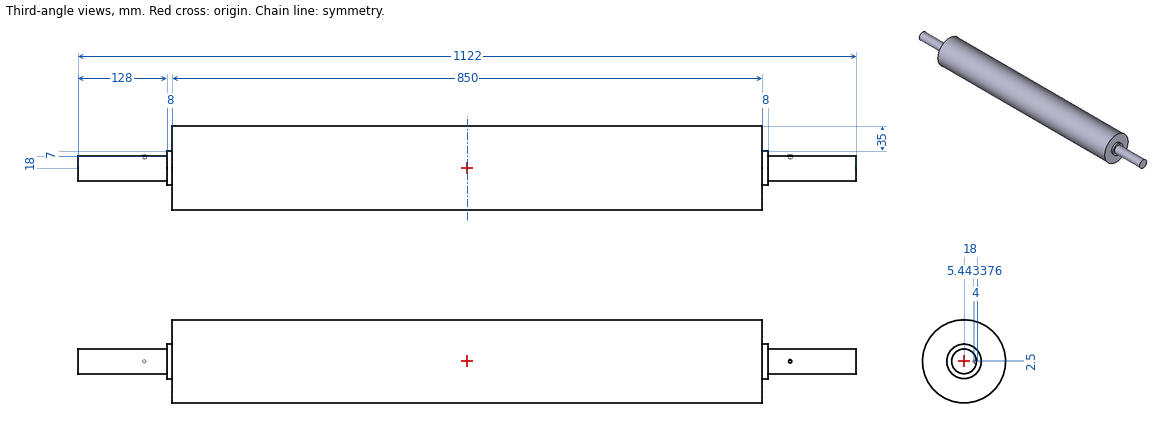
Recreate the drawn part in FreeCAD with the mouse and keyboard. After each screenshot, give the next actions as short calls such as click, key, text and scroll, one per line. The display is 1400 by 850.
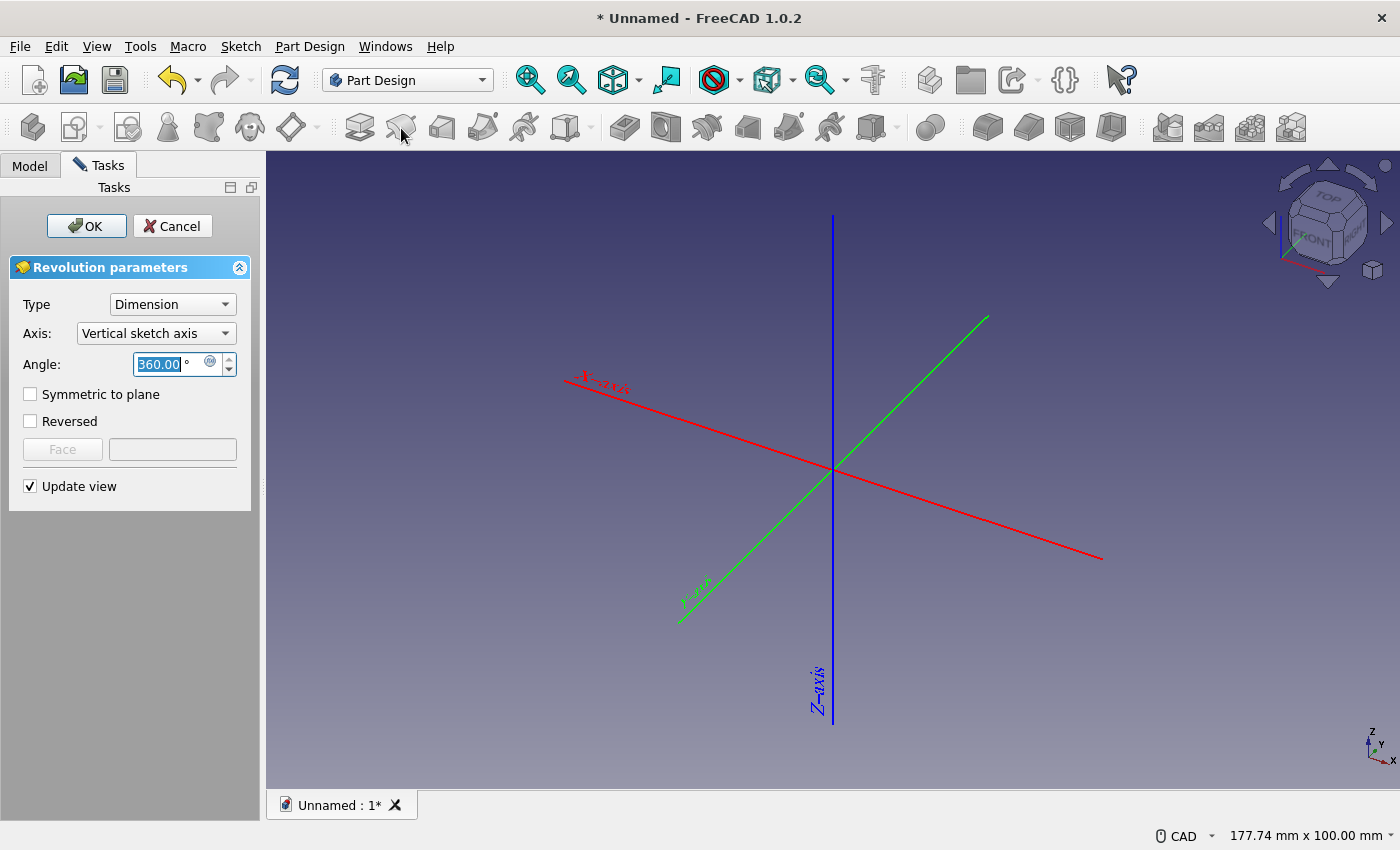
click(157, 334)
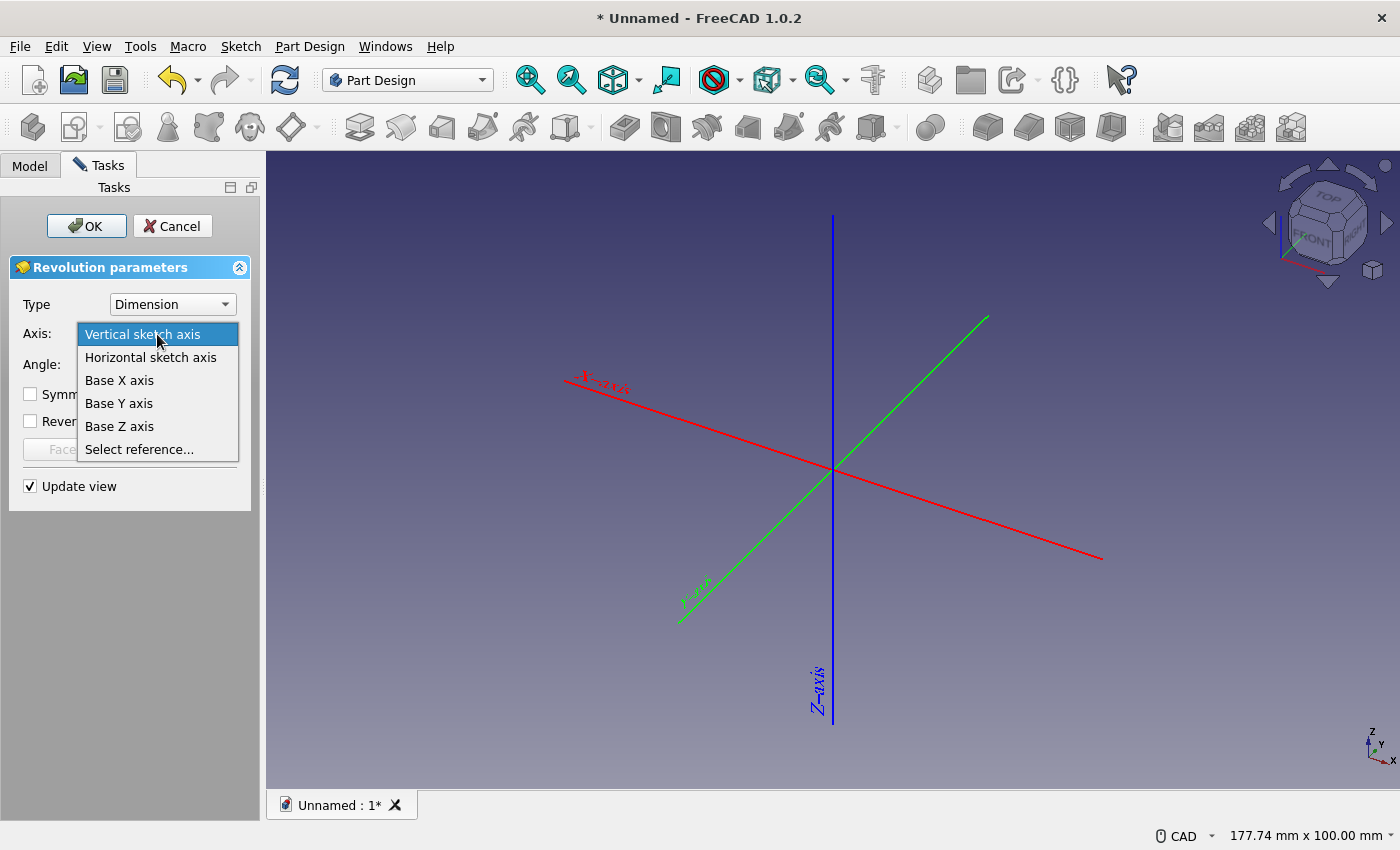
click(156, 358)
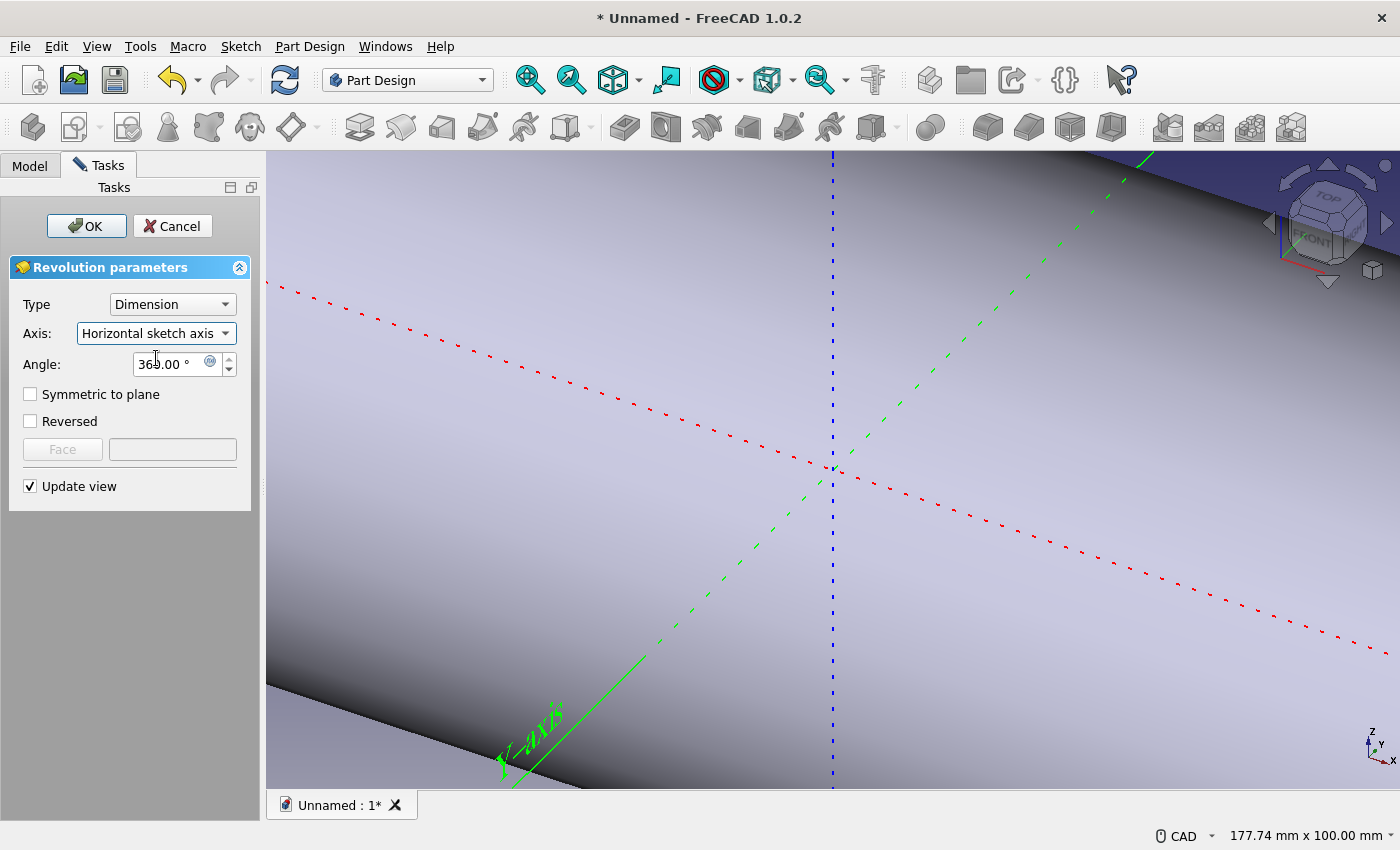
click(87, 226)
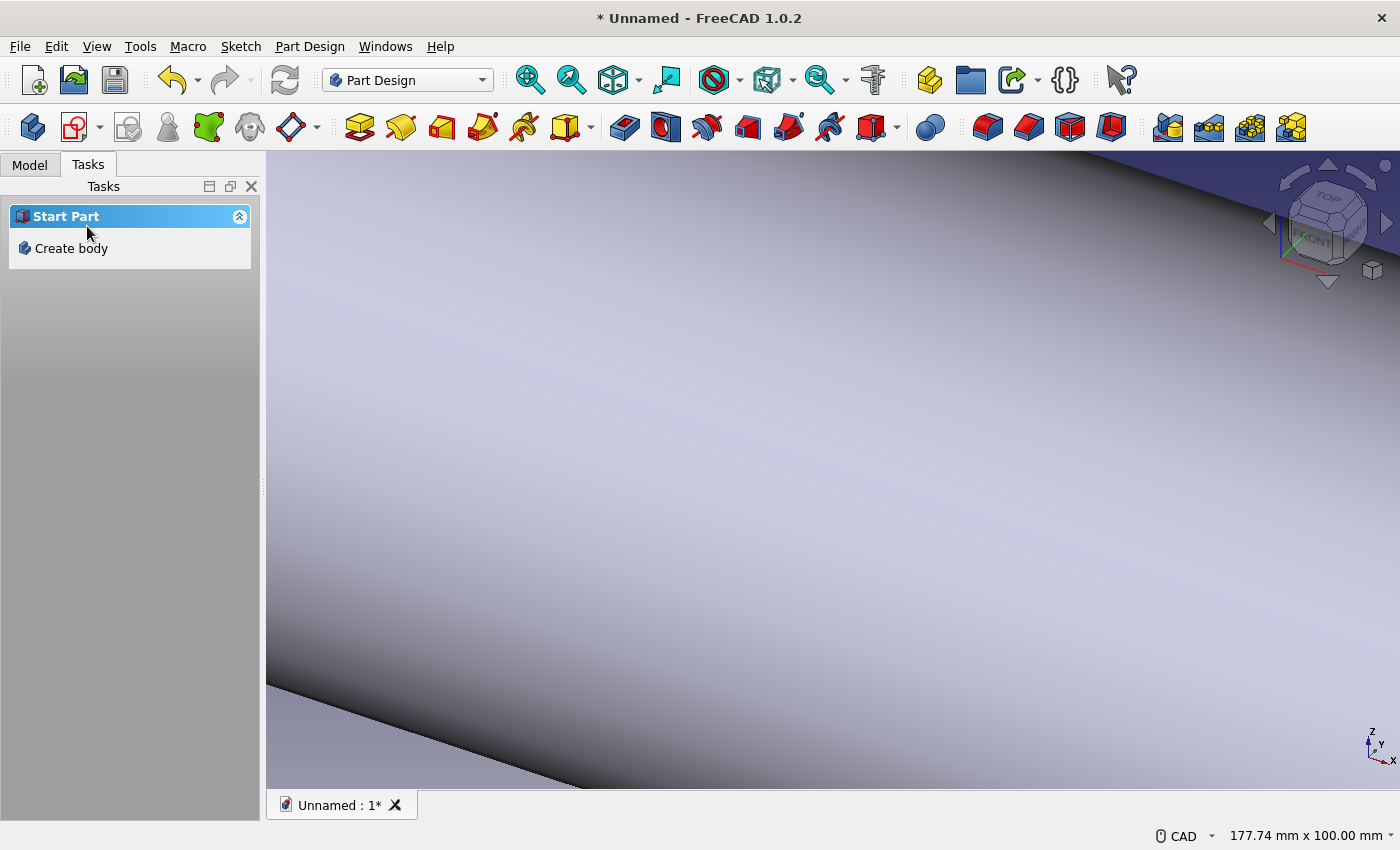
click(531, 80)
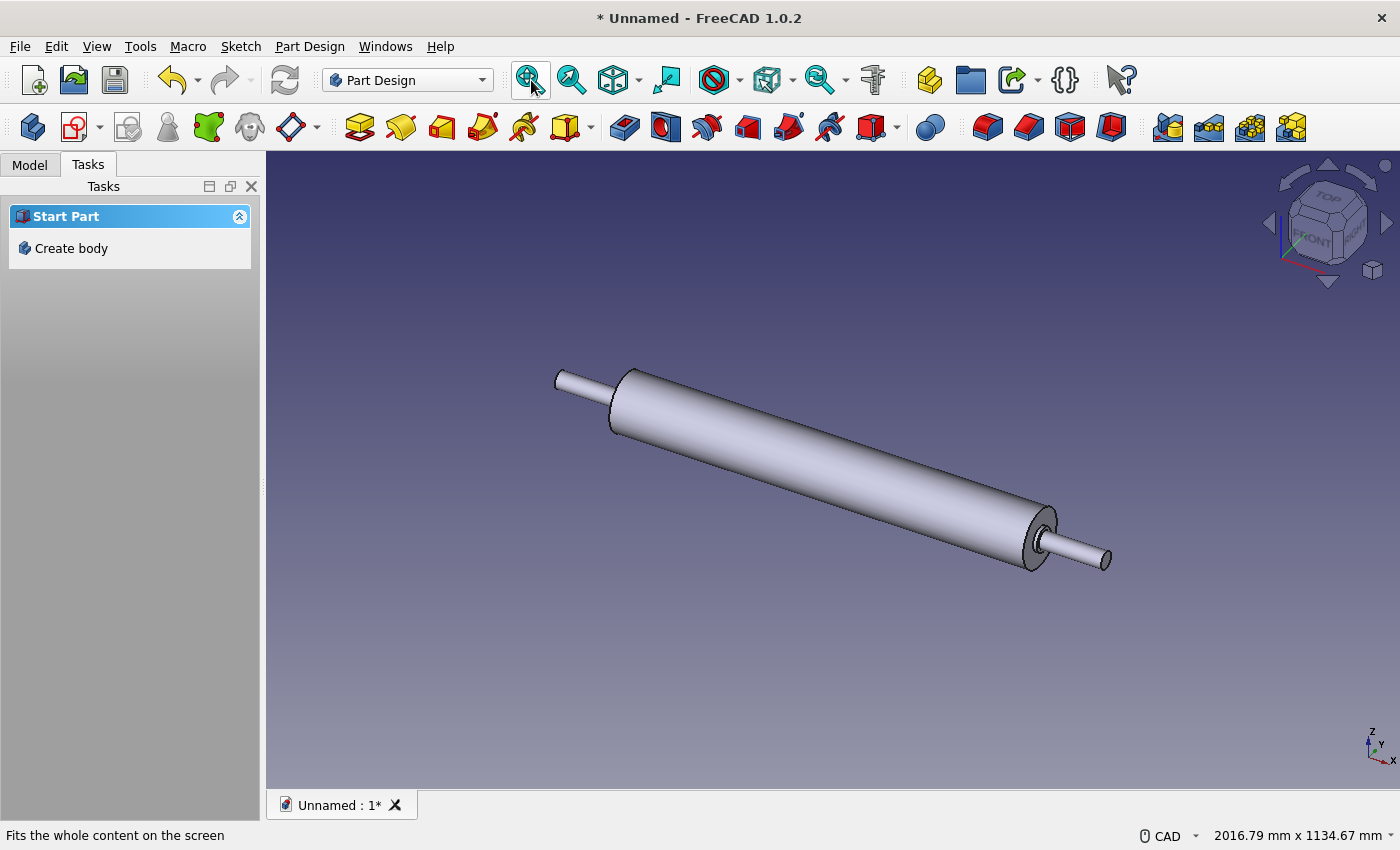
click(30, 164)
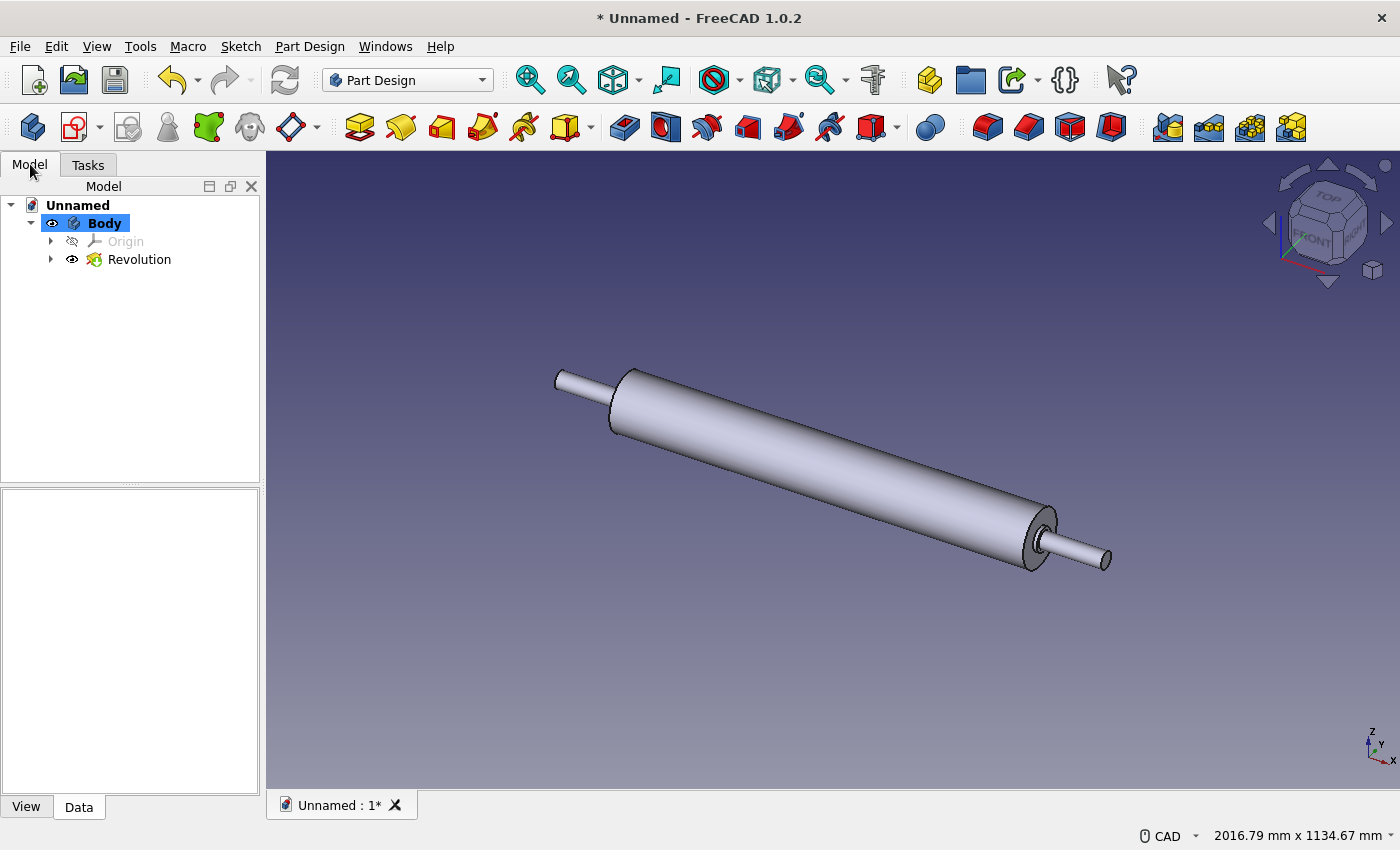
click(51, 241)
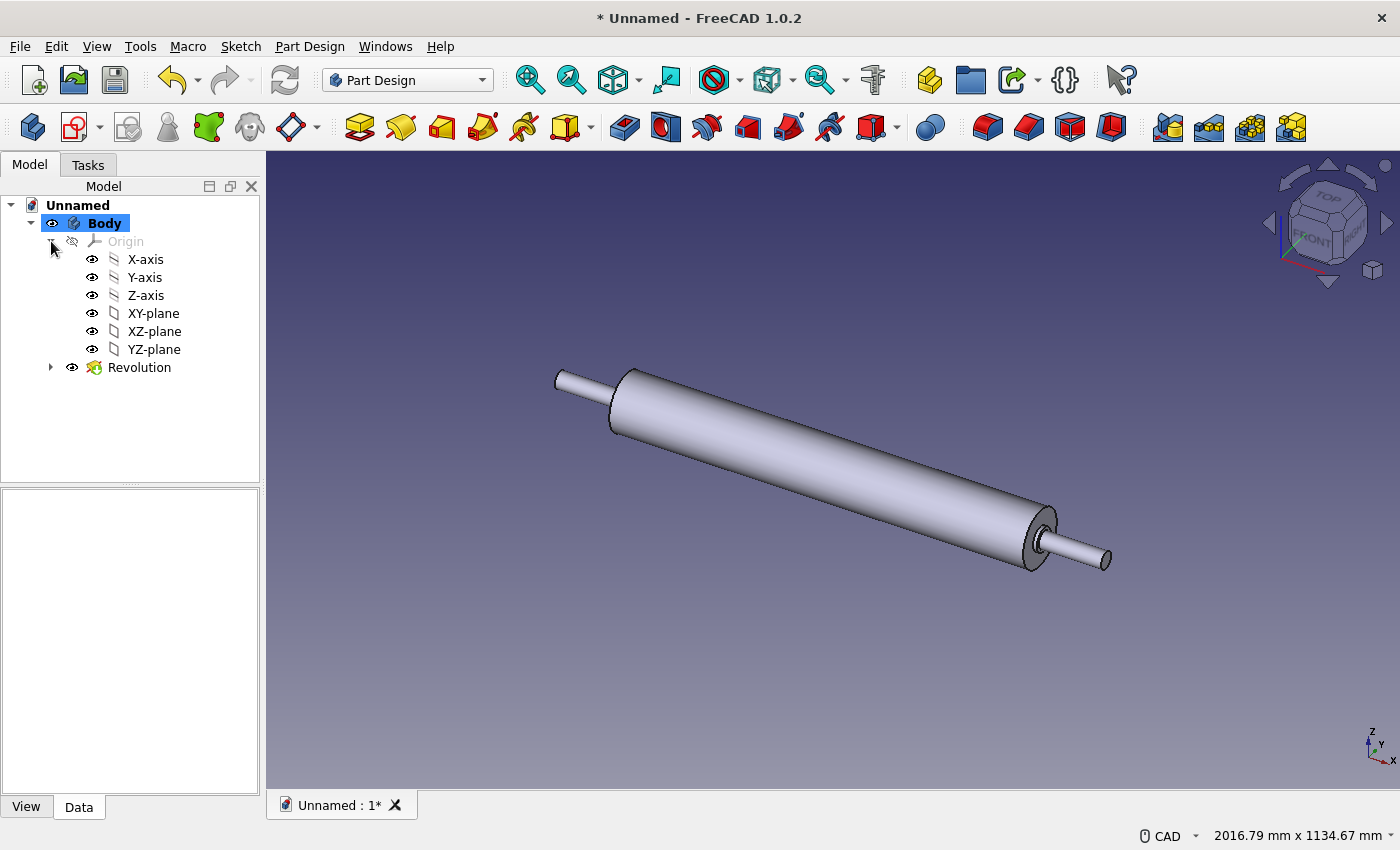
click(137, 349)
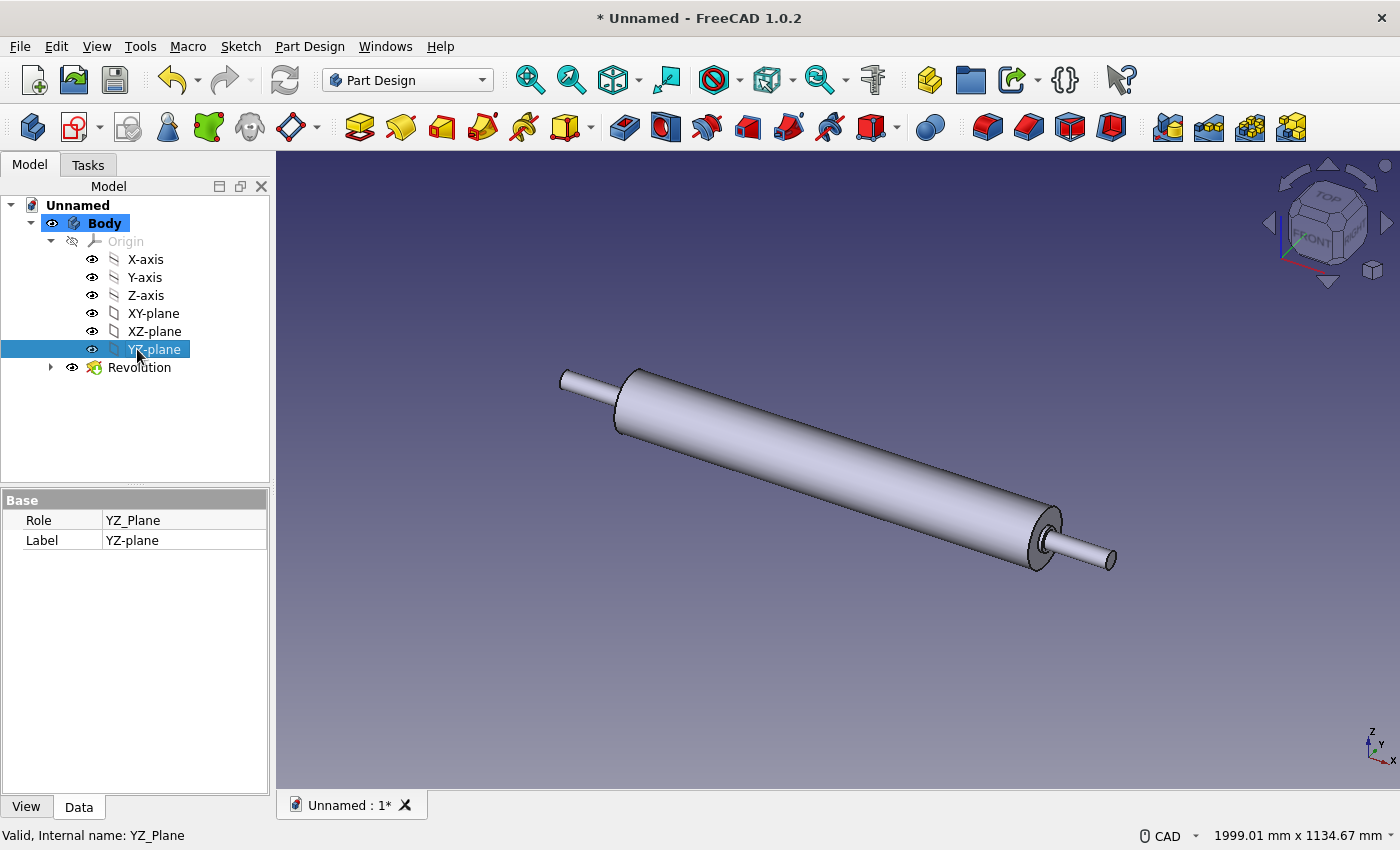
click(290, 128)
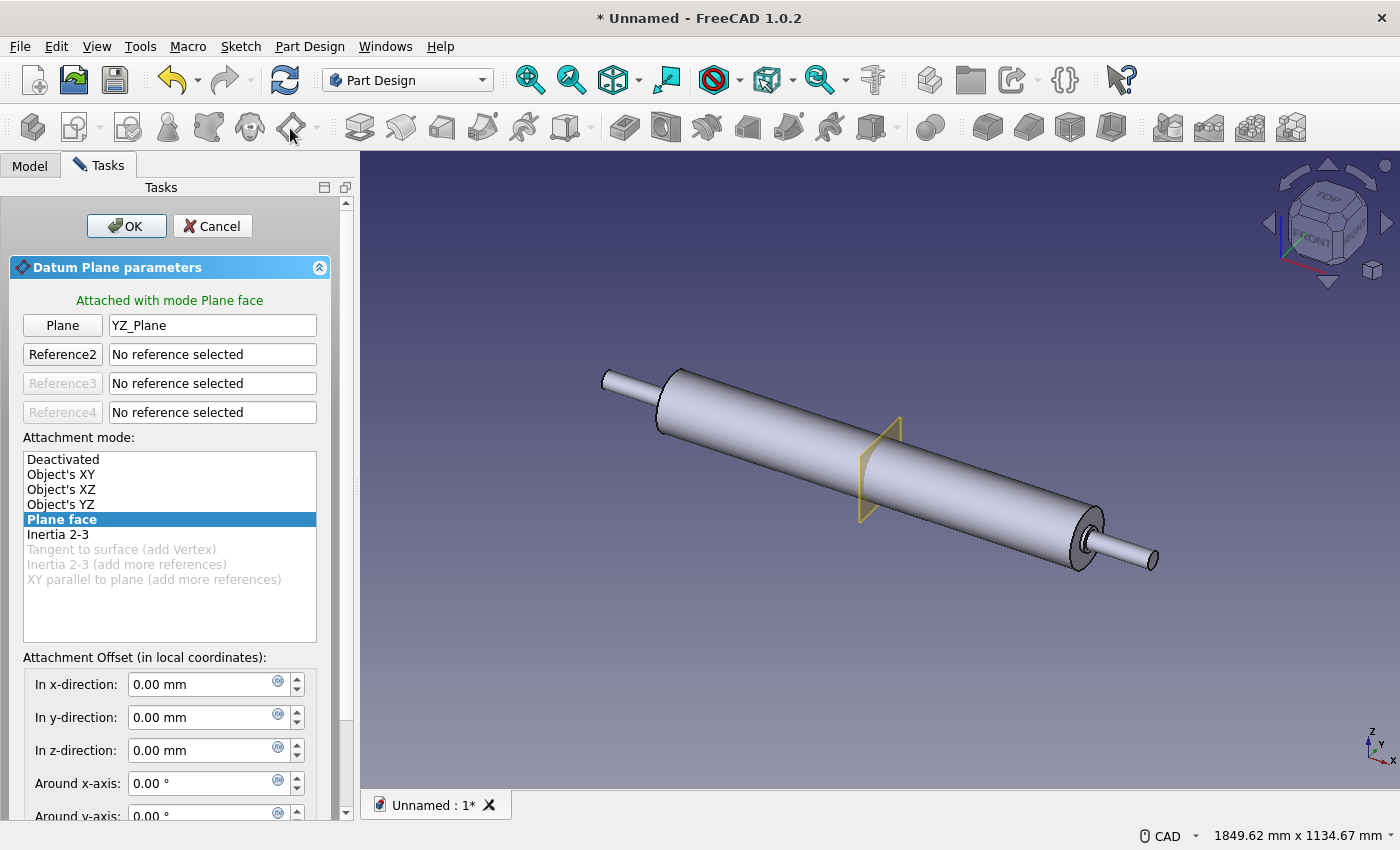
triple_click(210, 750)